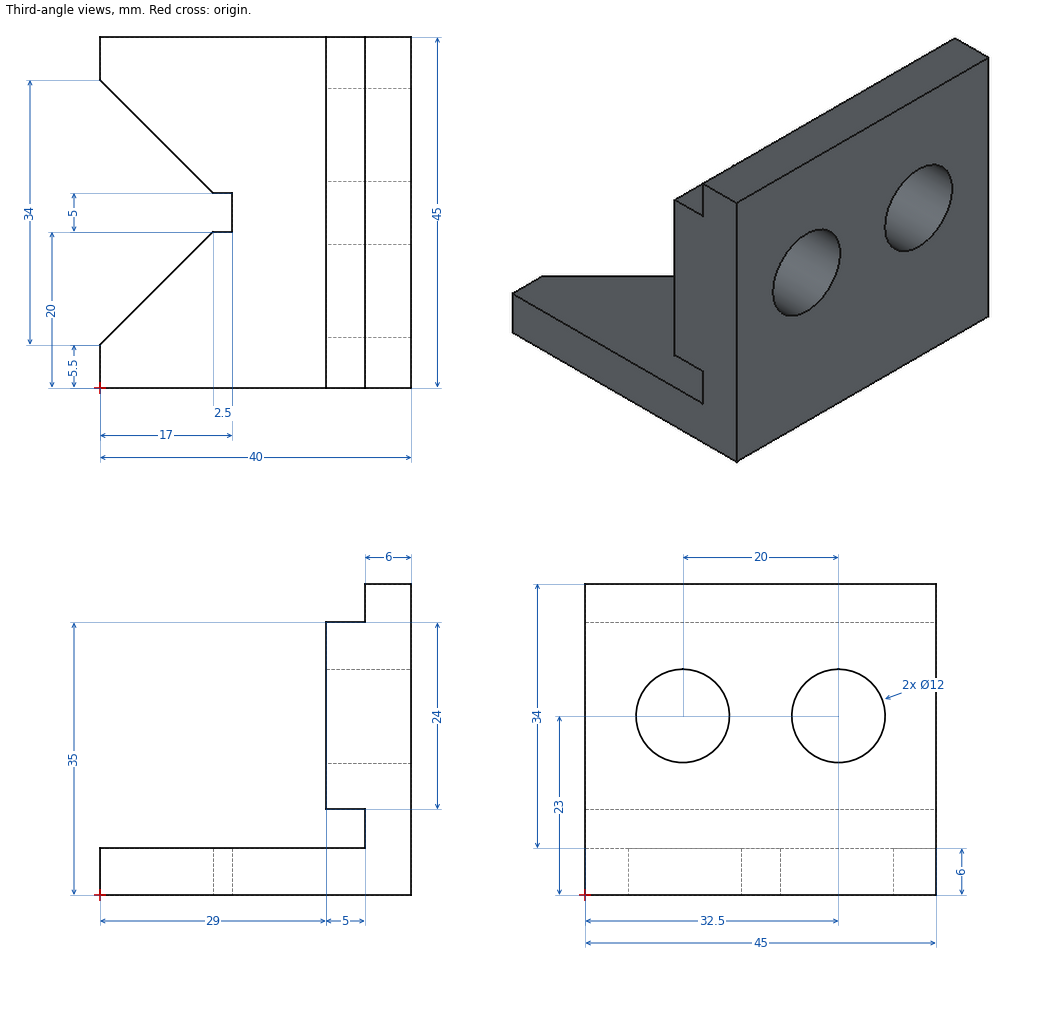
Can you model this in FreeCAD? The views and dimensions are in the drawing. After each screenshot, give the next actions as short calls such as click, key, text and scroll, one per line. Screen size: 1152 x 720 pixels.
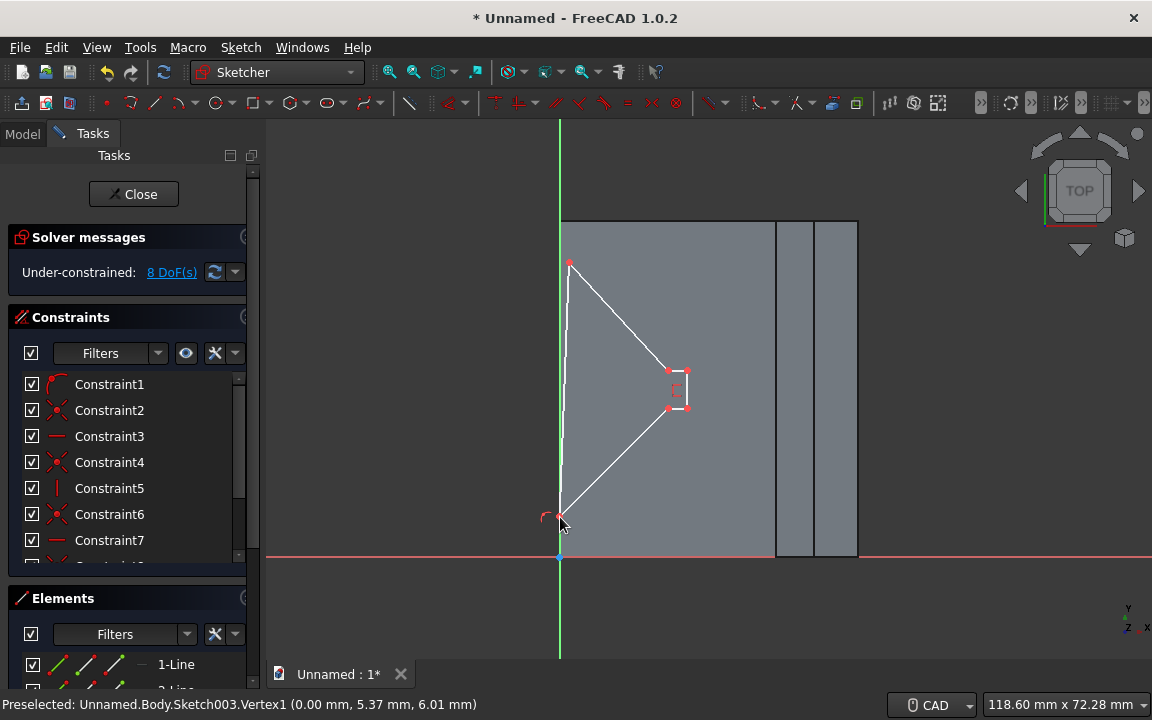
click(562, 441)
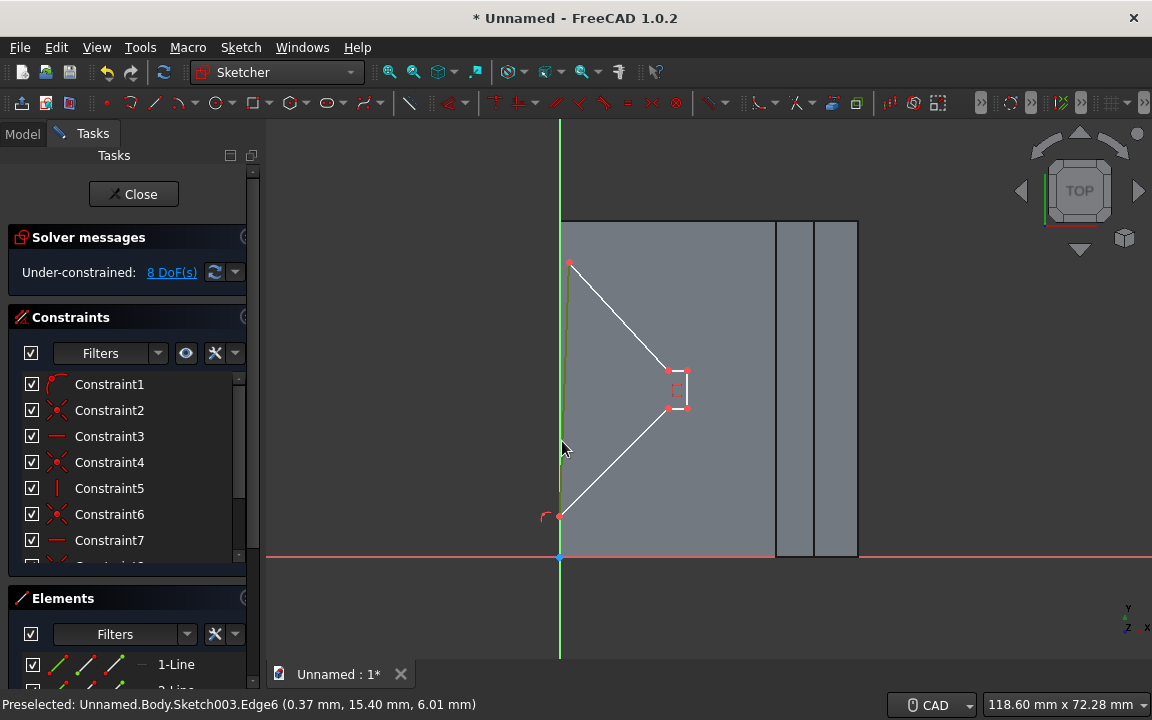
click(538, 104)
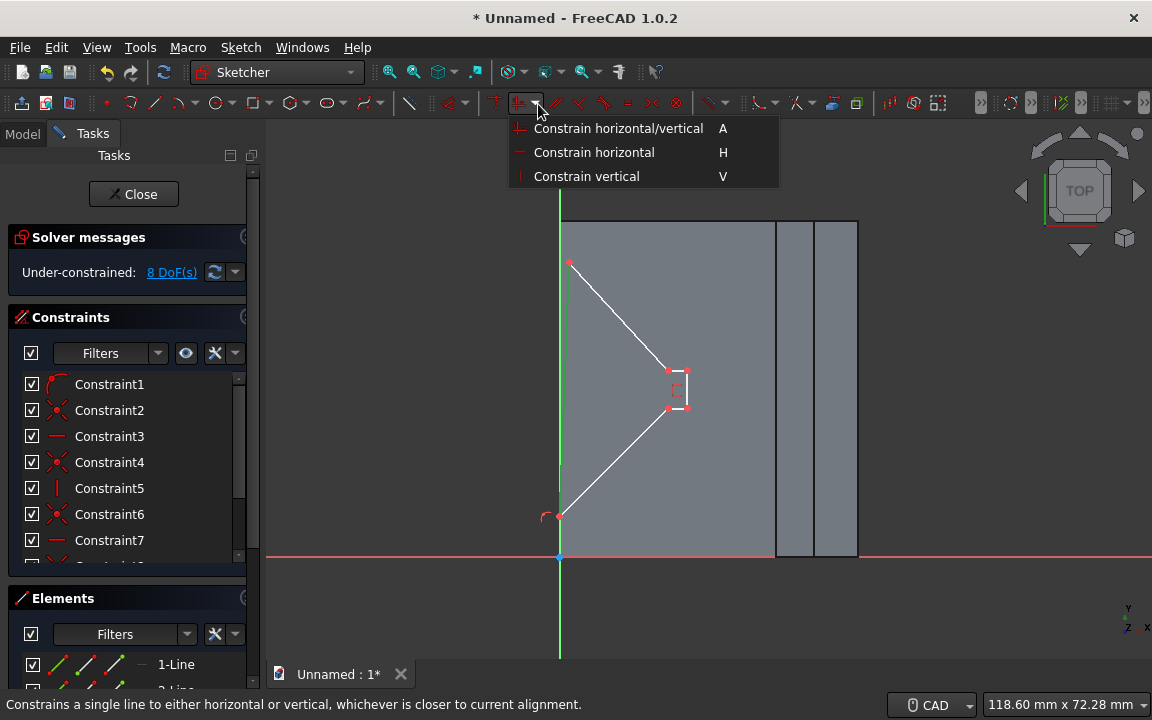
click(644, 176)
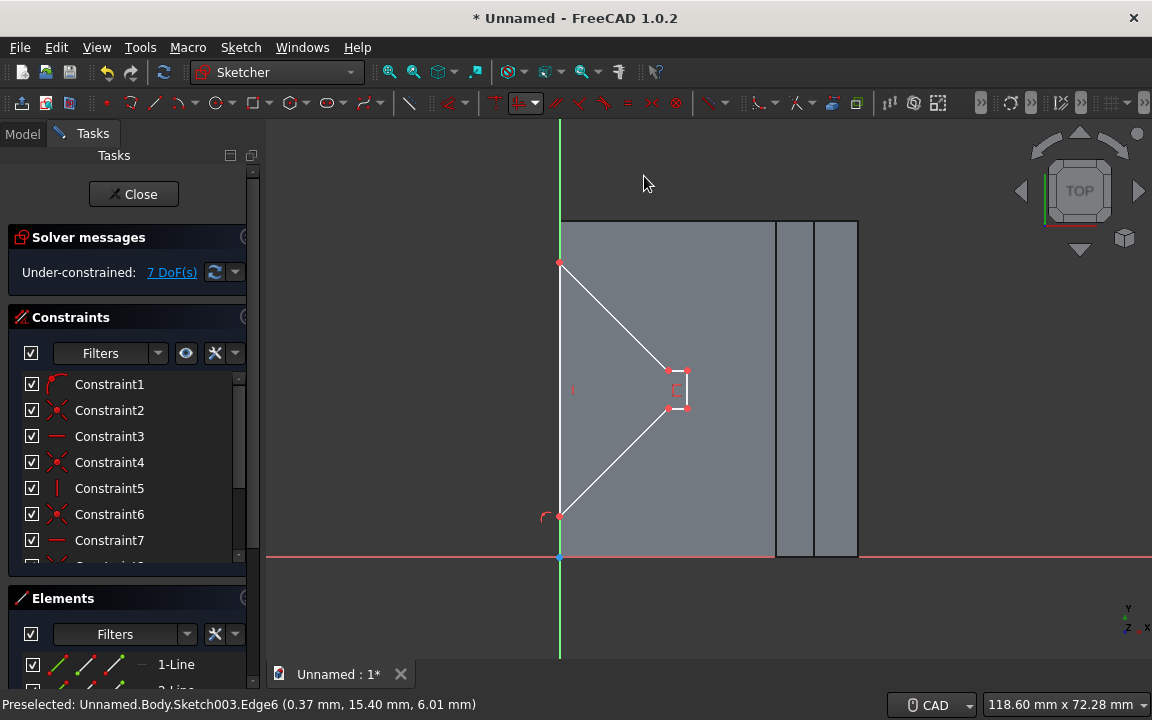
click(448, 104)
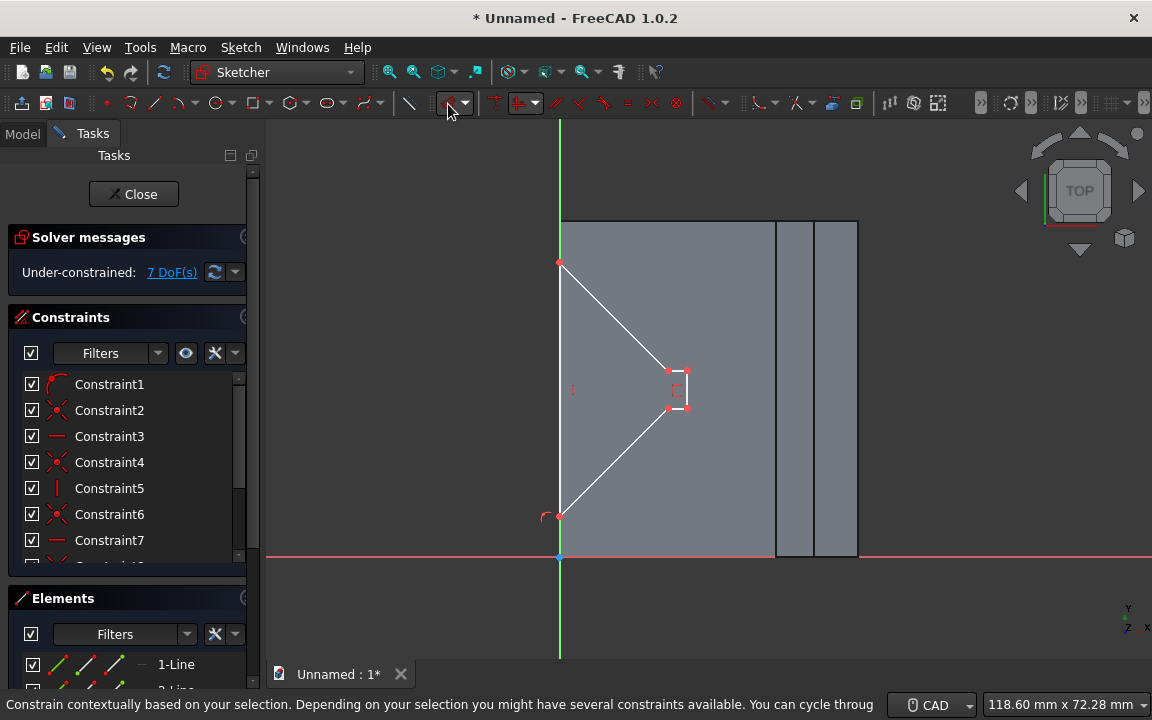
click(687, 398)
click(721, 390)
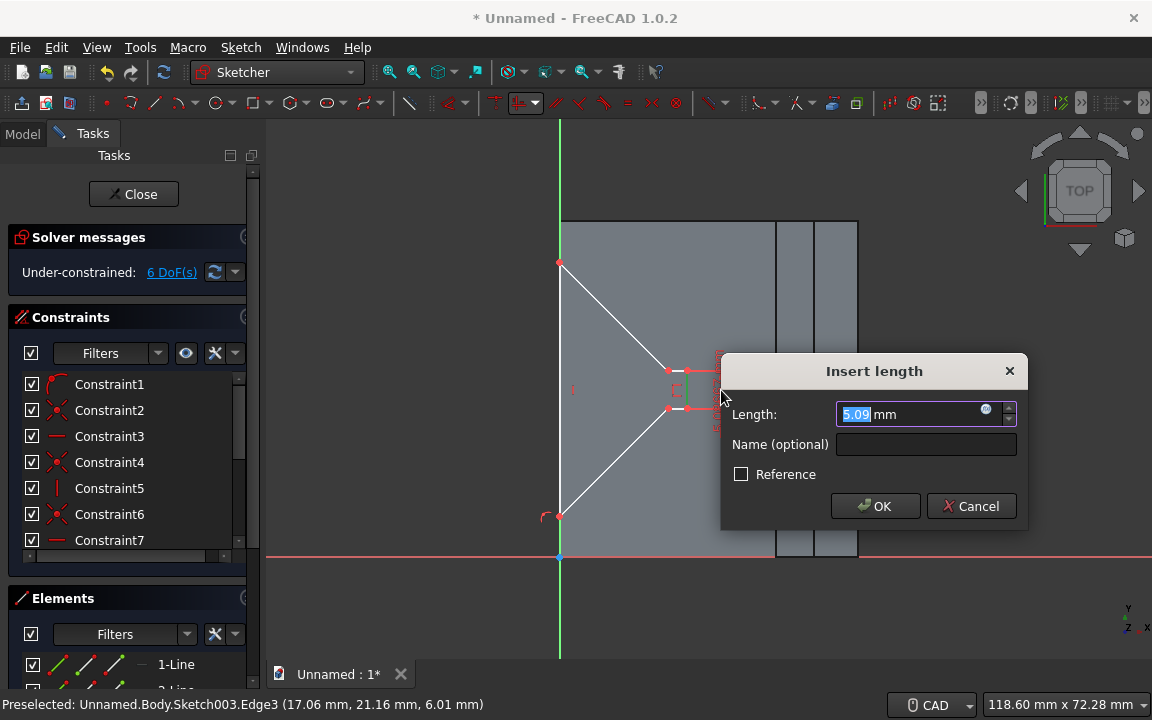
text(5)
key(Return)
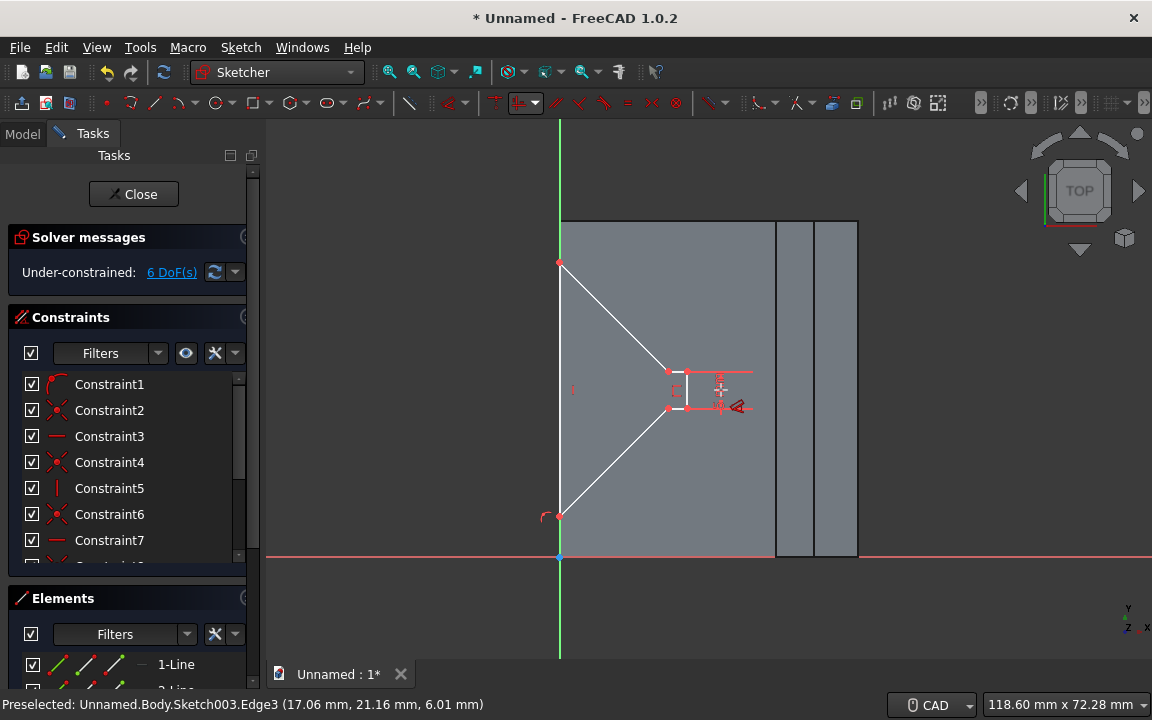
click(560, 339)
click(526, 390)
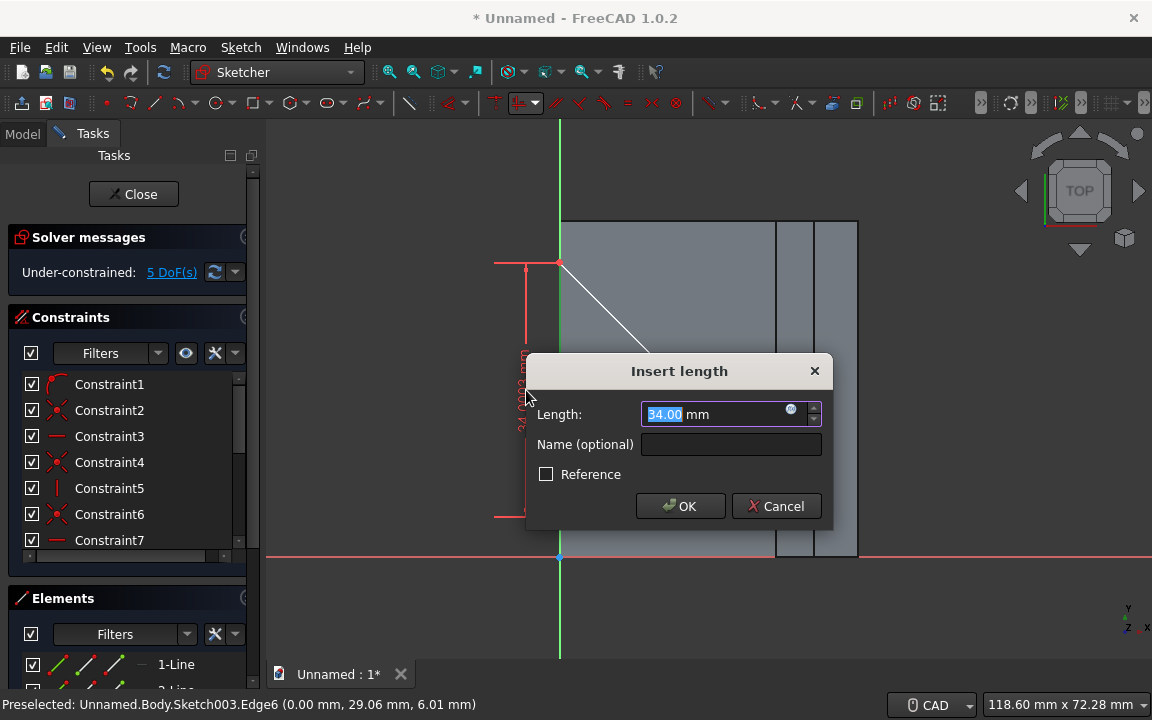
text(34)
key(Return)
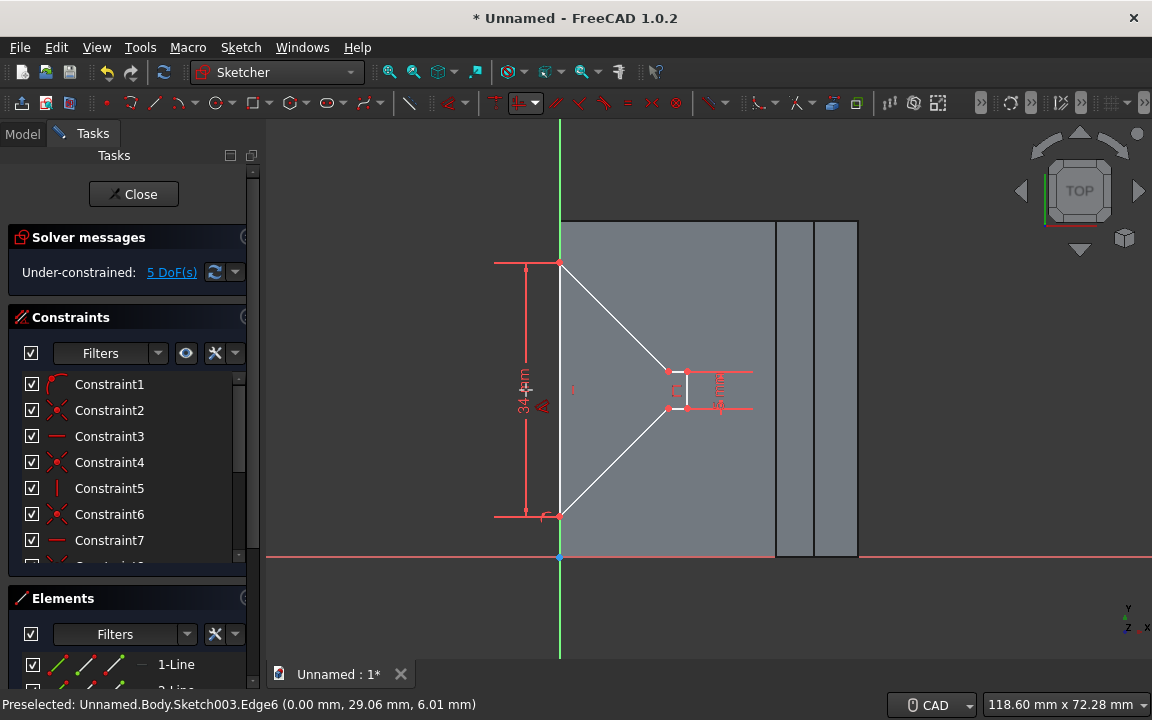
scroll(677, 409, up, 4)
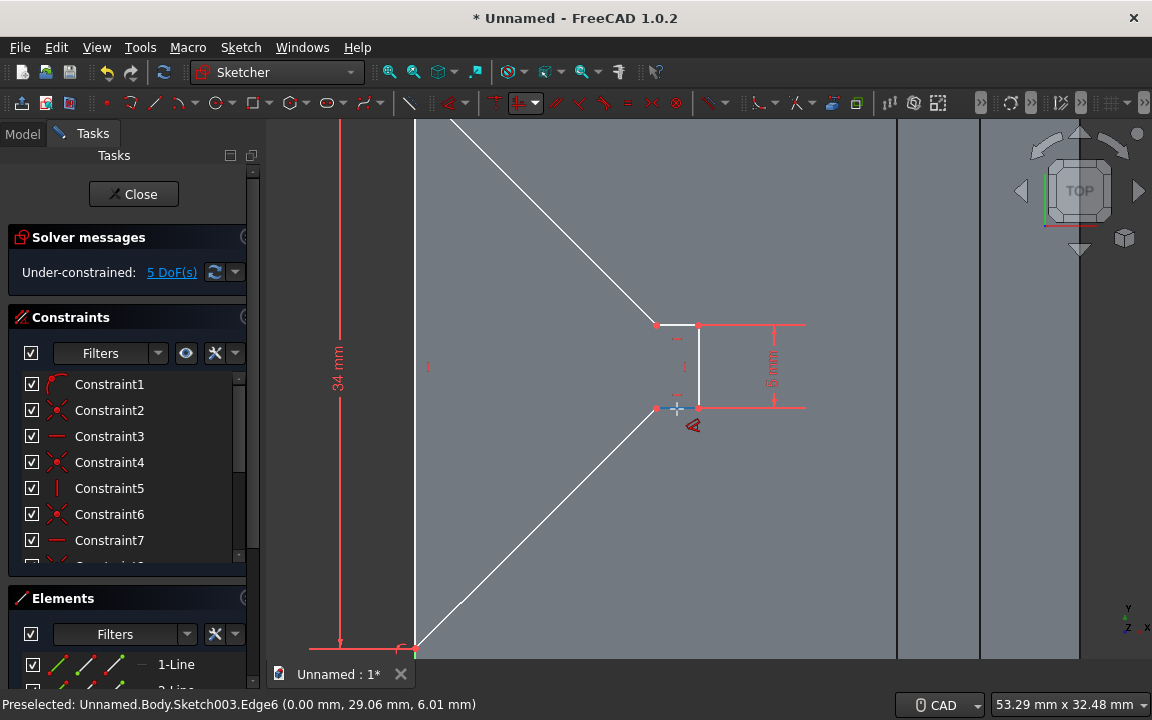
click(678, 408)
click(678, 374)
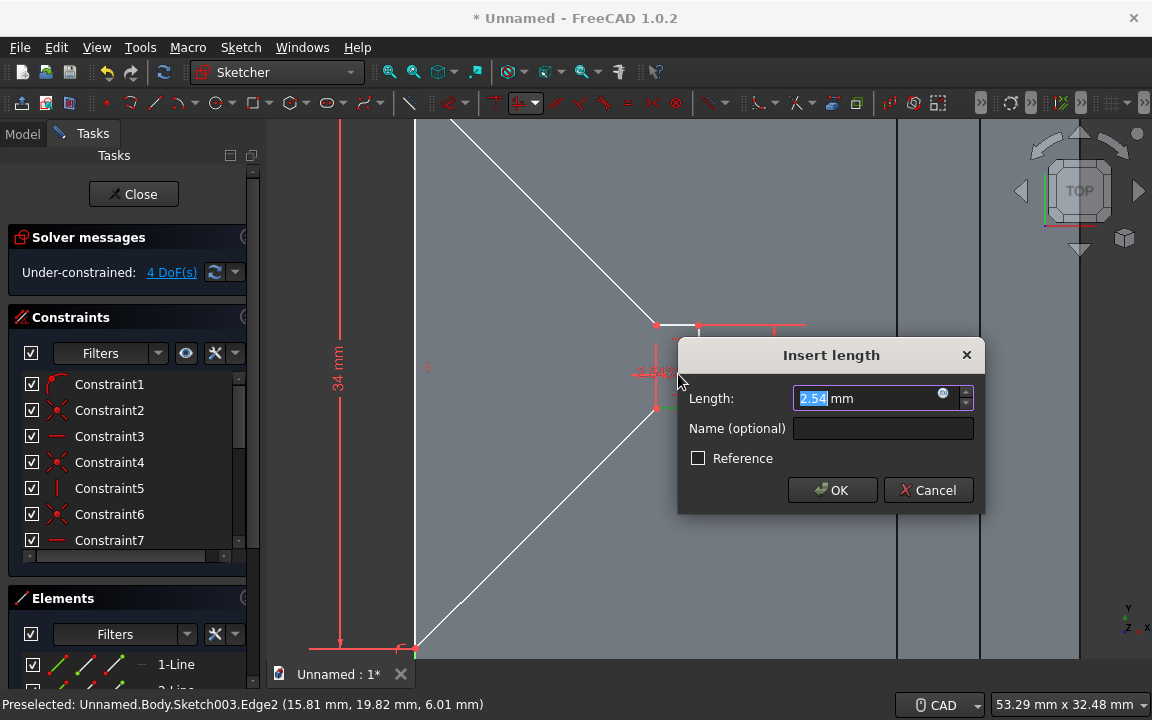
text(2.5)
key(Return)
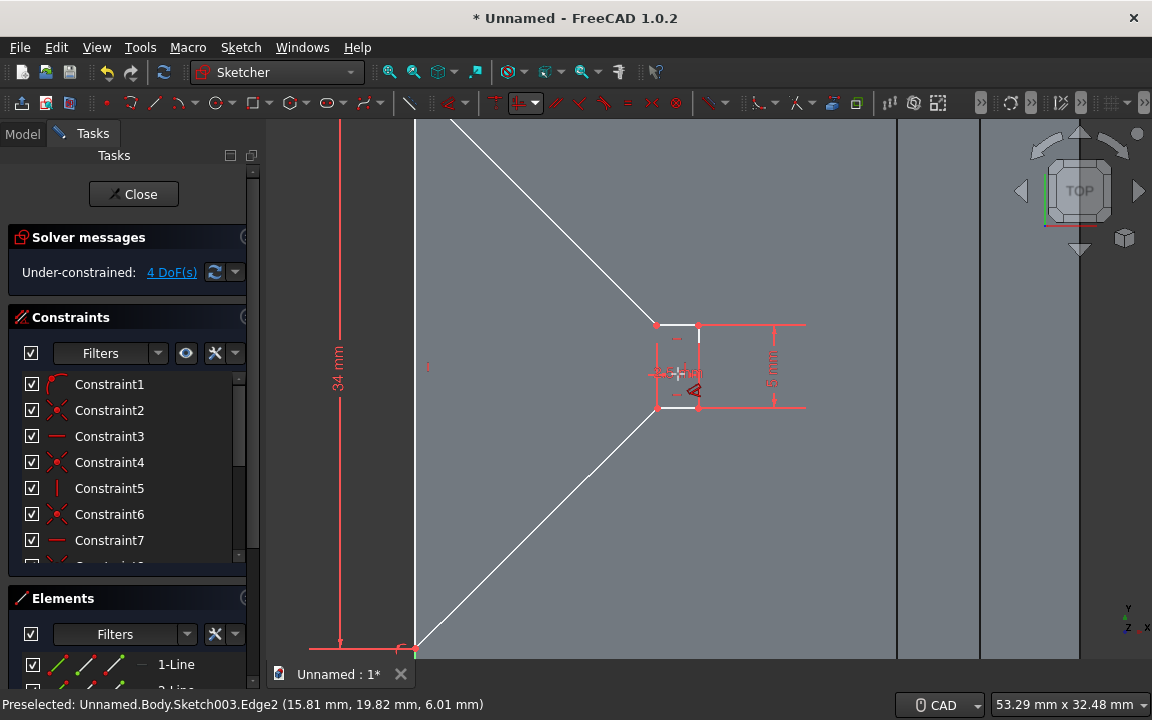
click(686, 325)
click(678, 291)